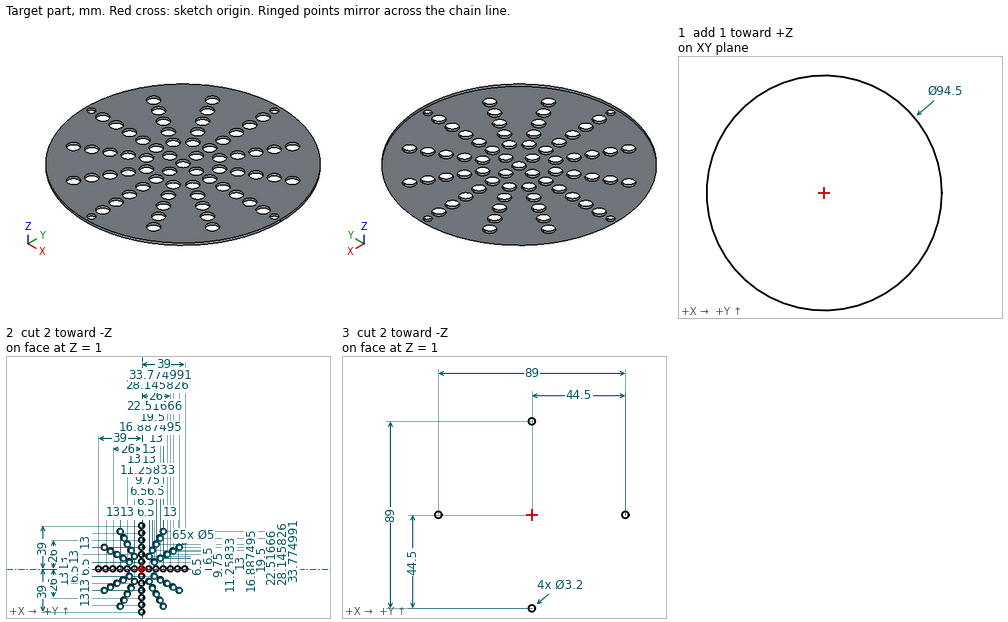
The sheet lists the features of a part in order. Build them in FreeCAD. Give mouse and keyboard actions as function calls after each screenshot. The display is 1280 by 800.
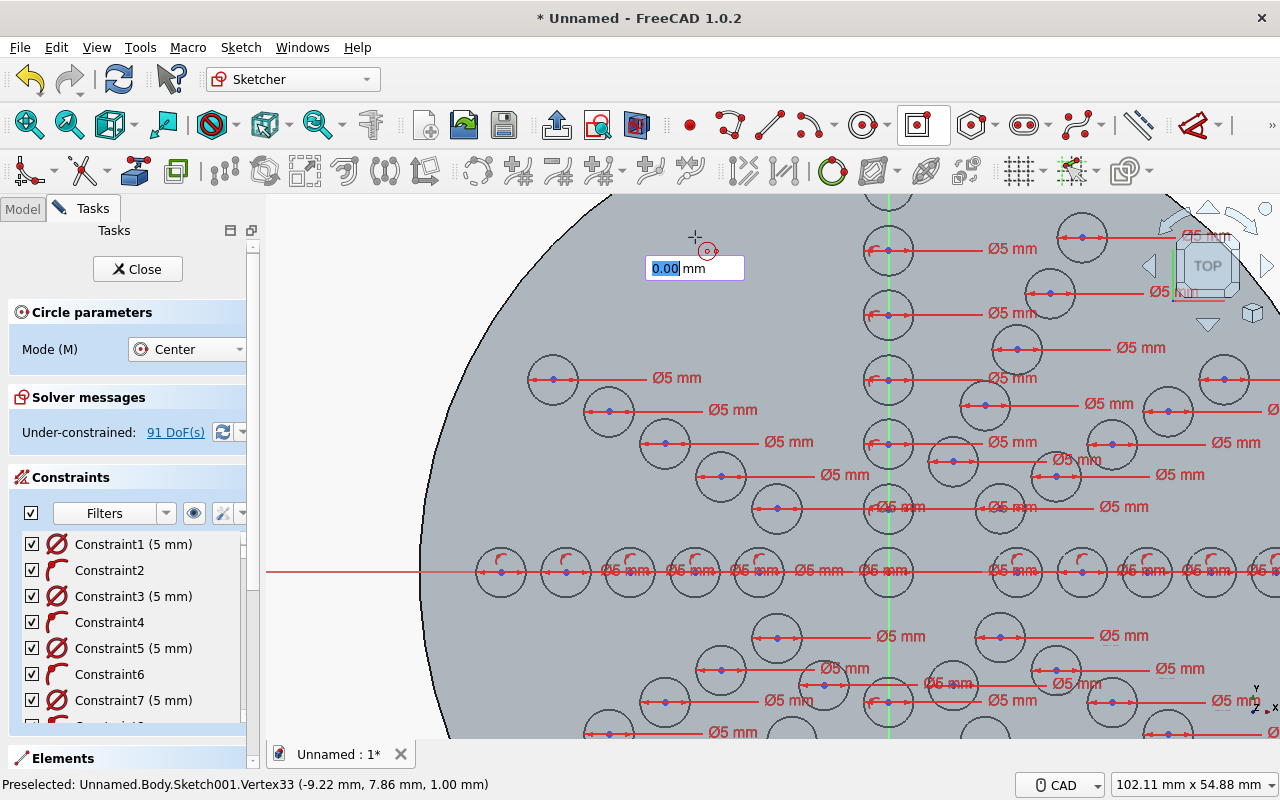
scroll(554, 380, down, 4)
move(625, 308)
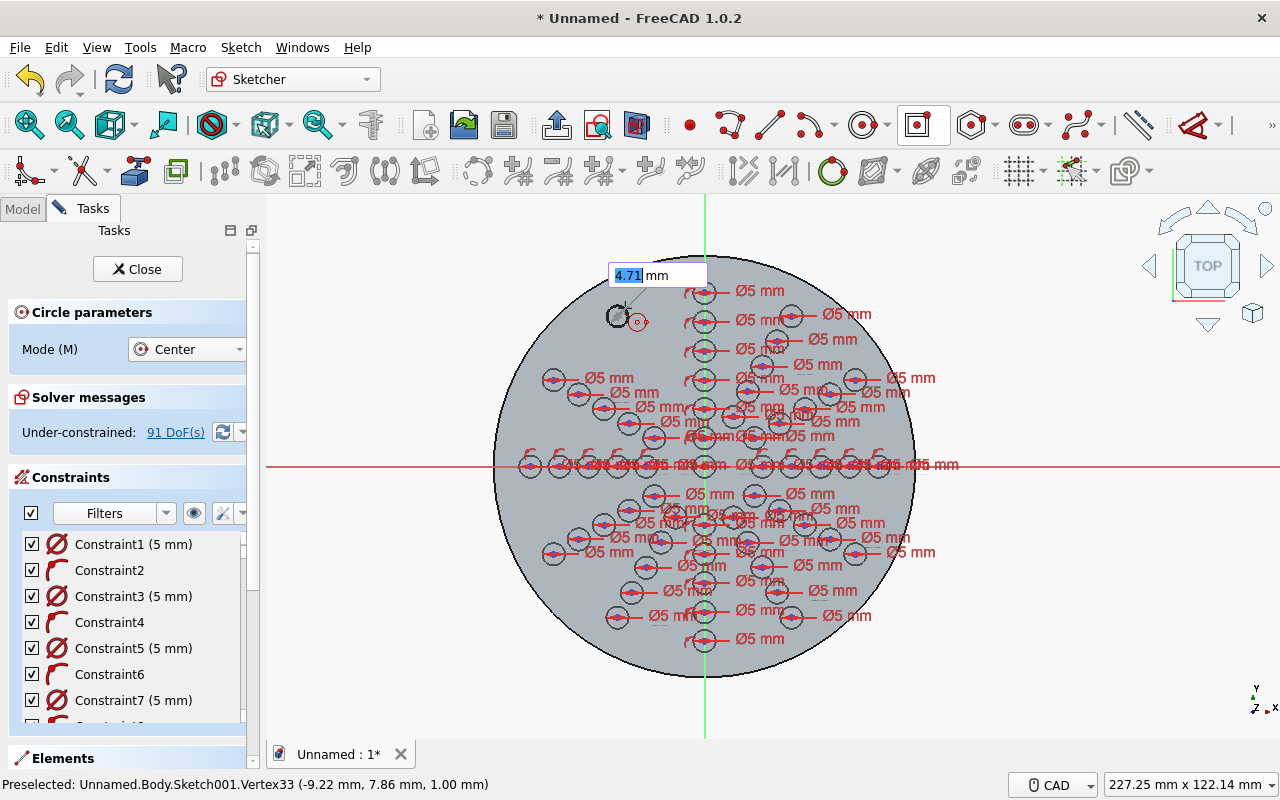
text(5)
key(Return)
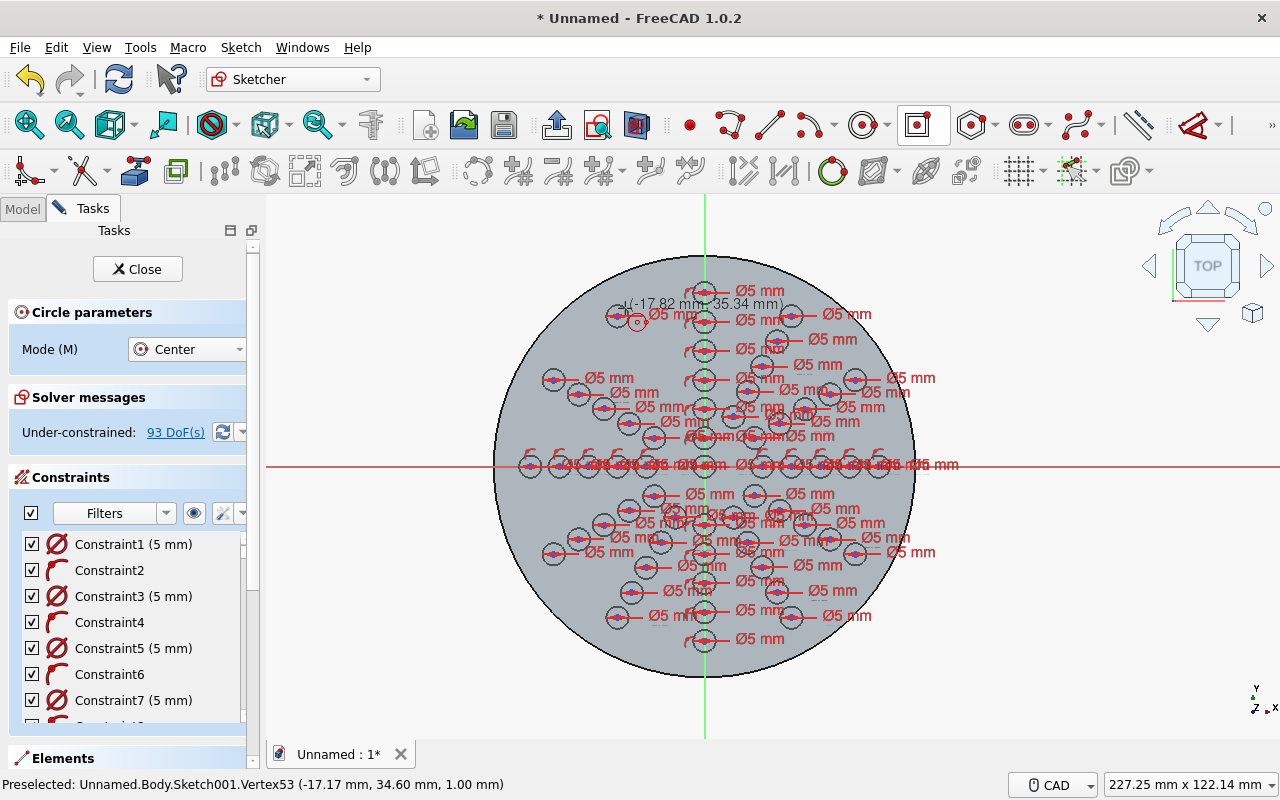
scroll(632, 341, up, 4)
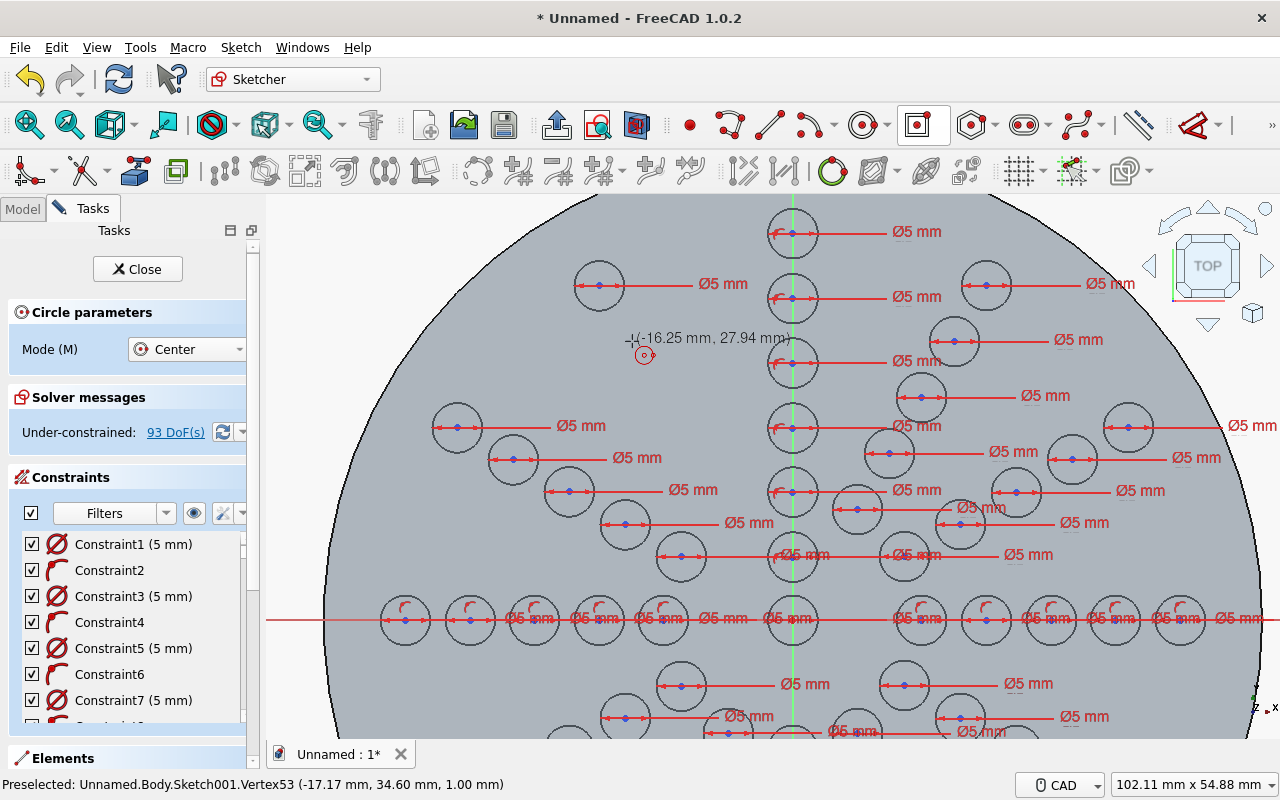
click(632, 341)
move(649, 323)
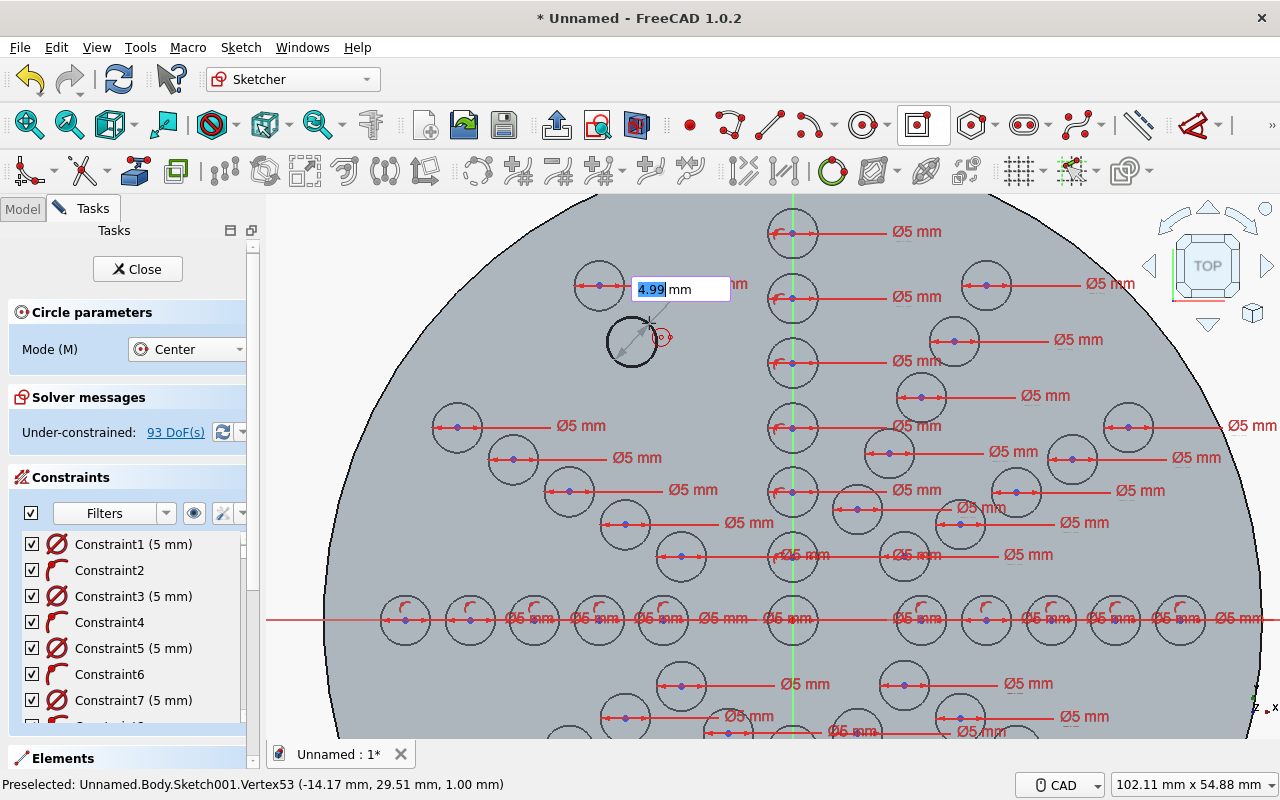
text(5)
key(Return)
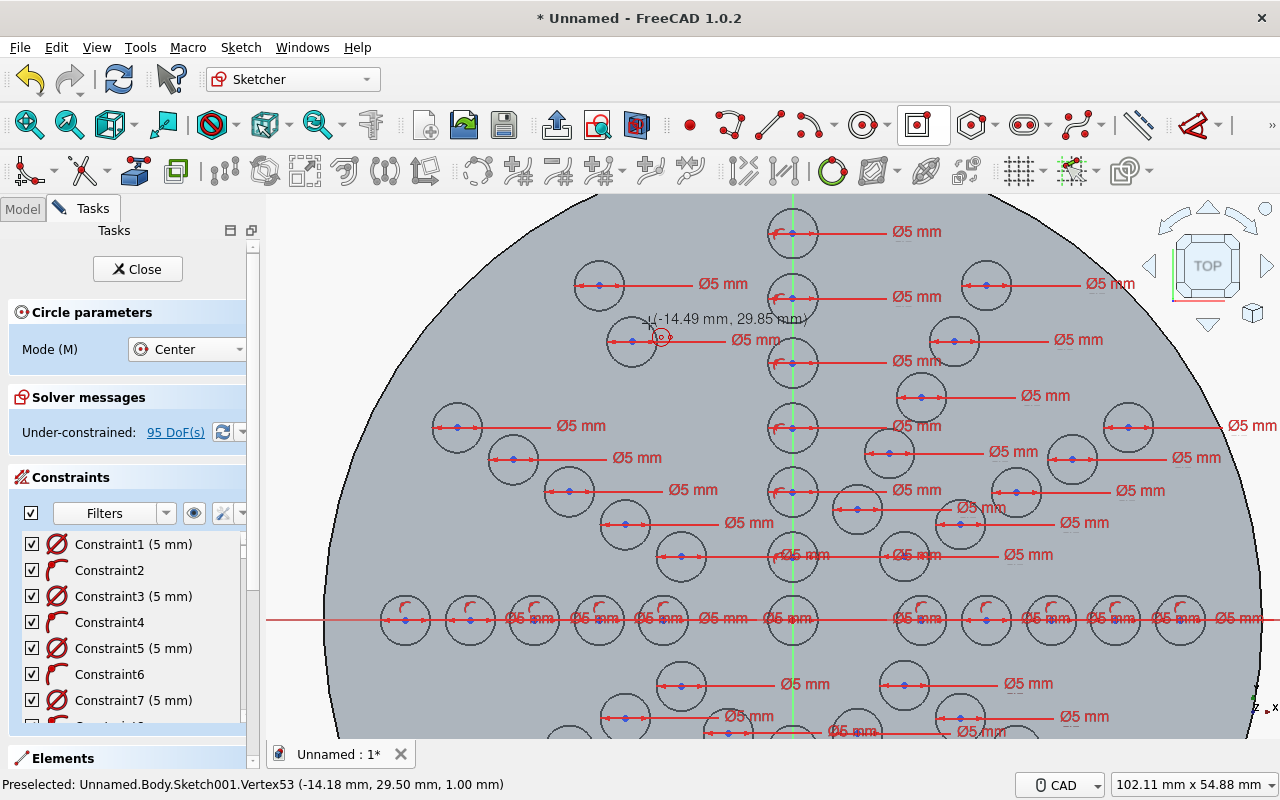
click(664, 397)
move(681, 379)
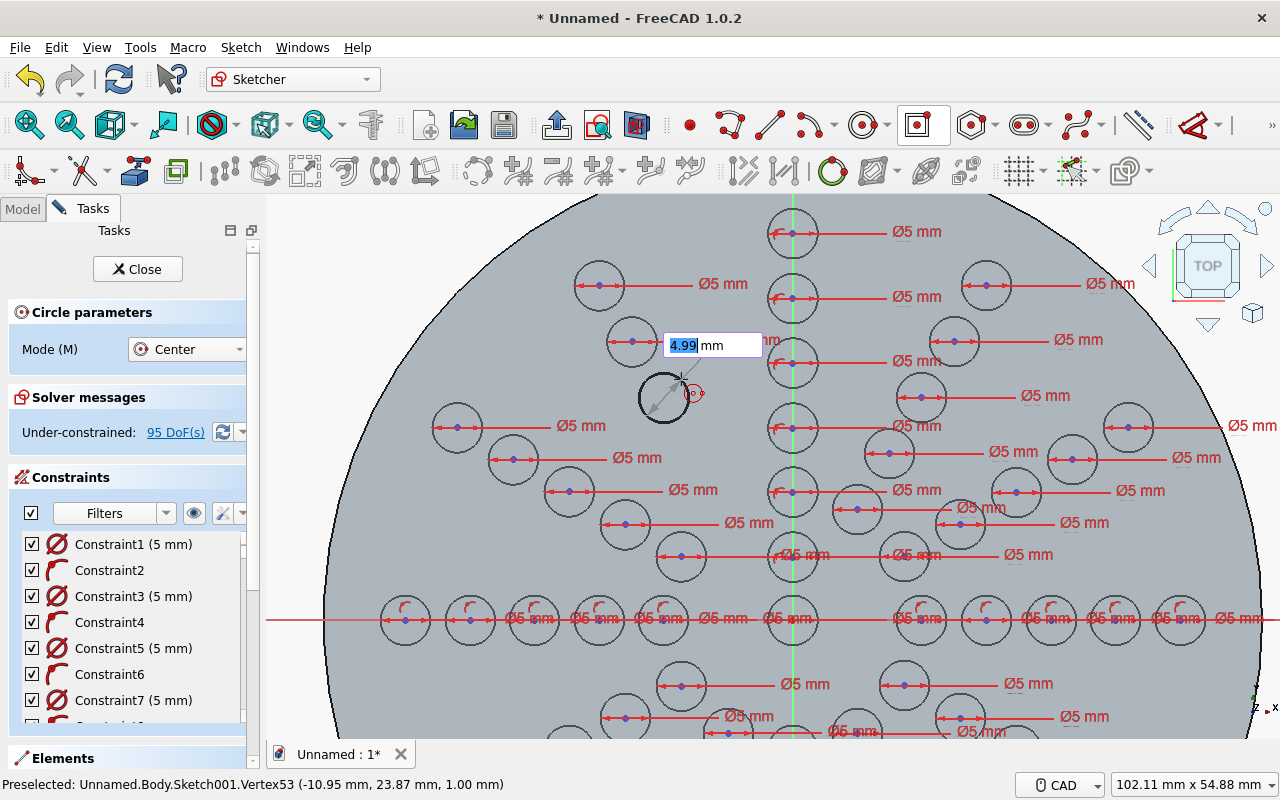
text(5)
key(Return)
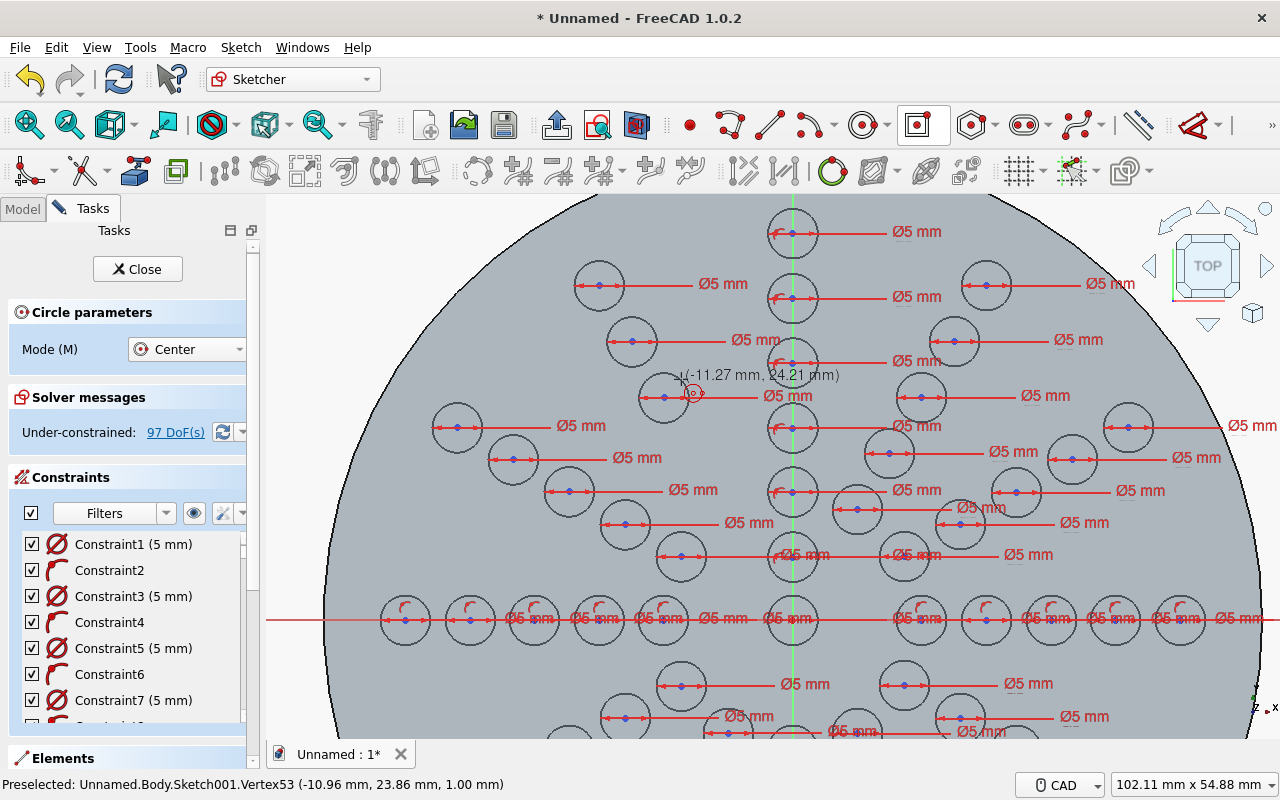
click(696, 453)
move(714, 435)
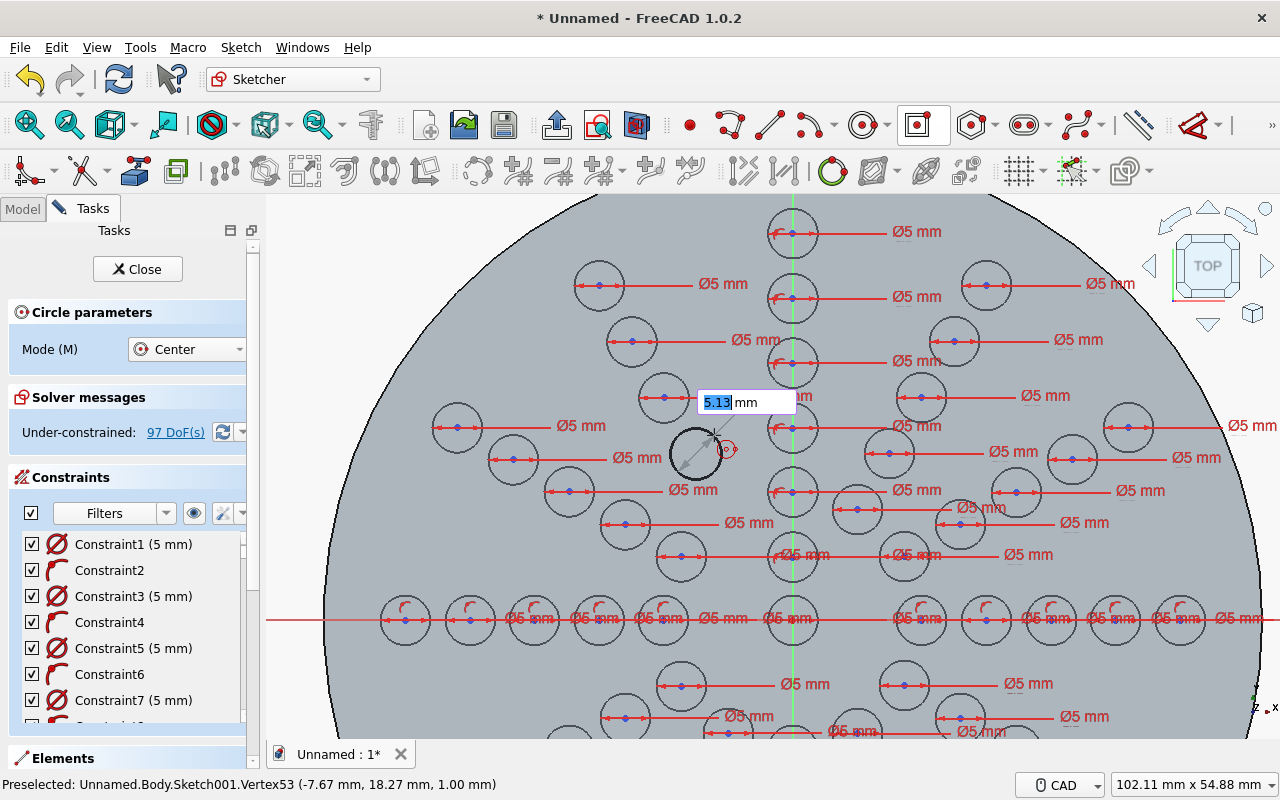
text(5)
key(Return)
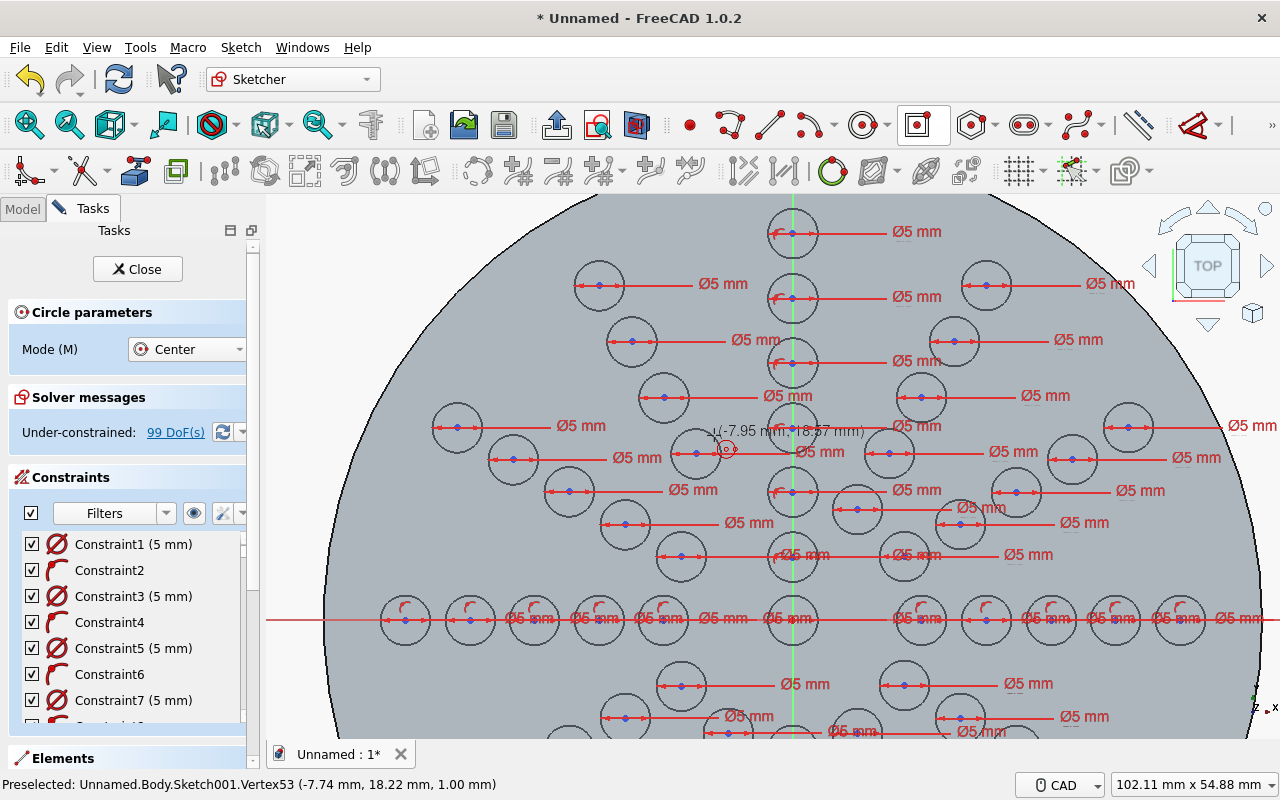
click(728, 509)
move(746, 491)